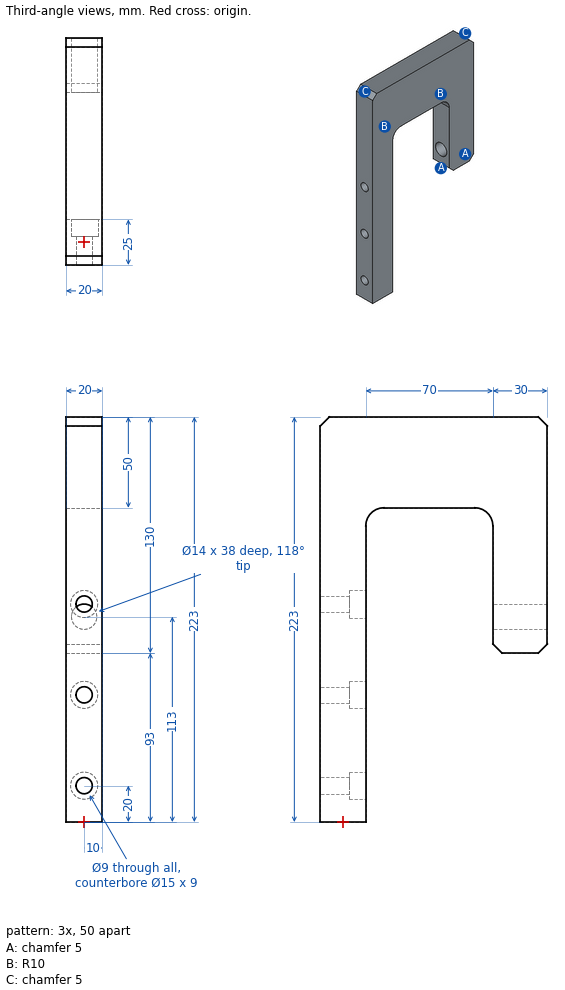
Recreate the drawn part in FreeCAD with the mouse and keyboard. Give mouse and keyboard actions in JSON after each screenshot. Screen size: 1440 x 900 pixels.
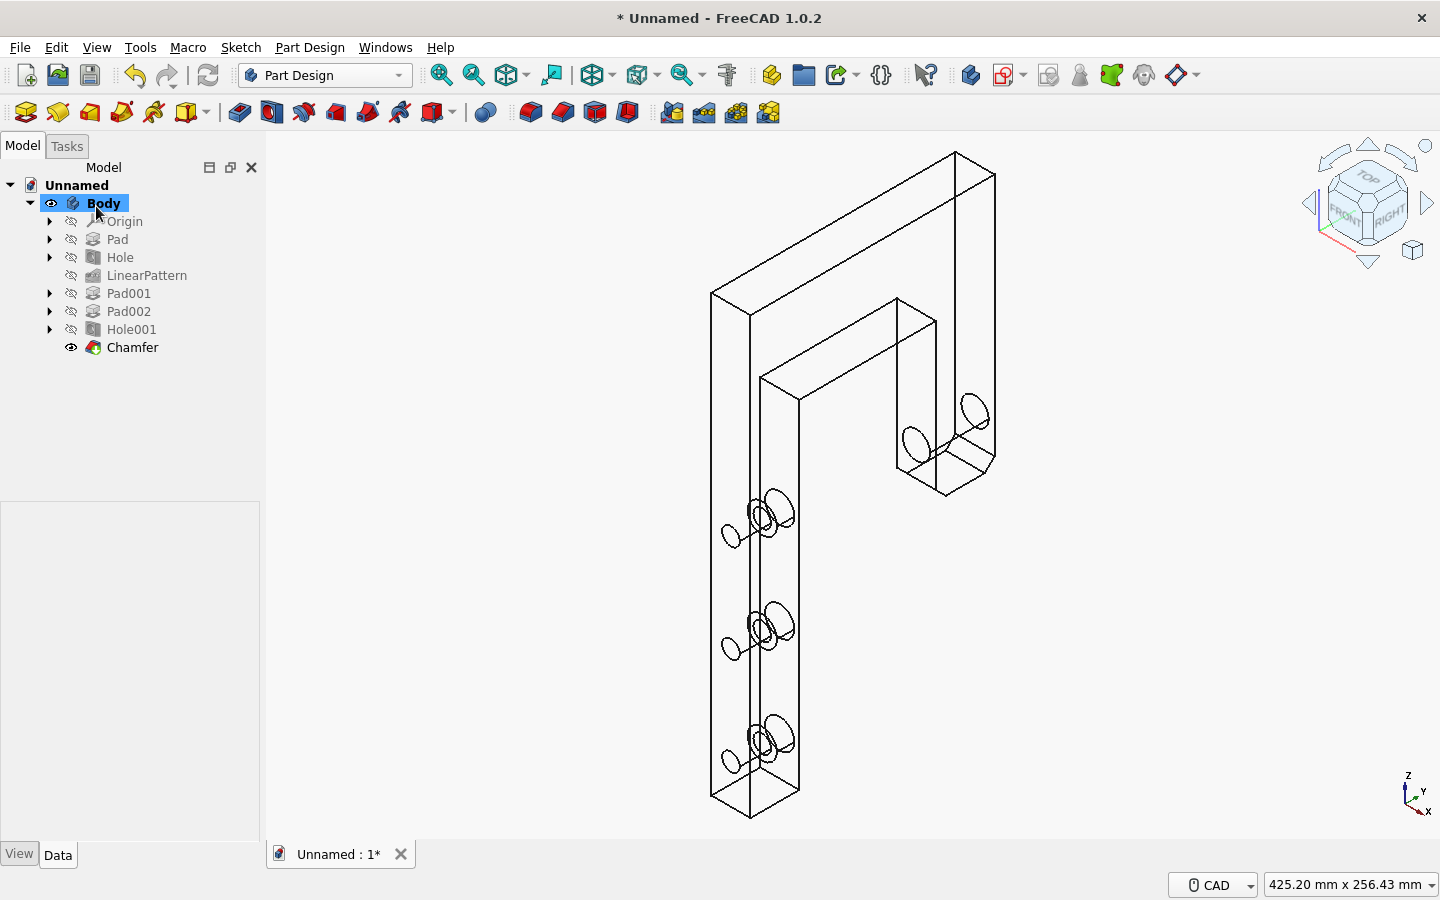
{"action": "left_click", "coordinate": [780, 388]}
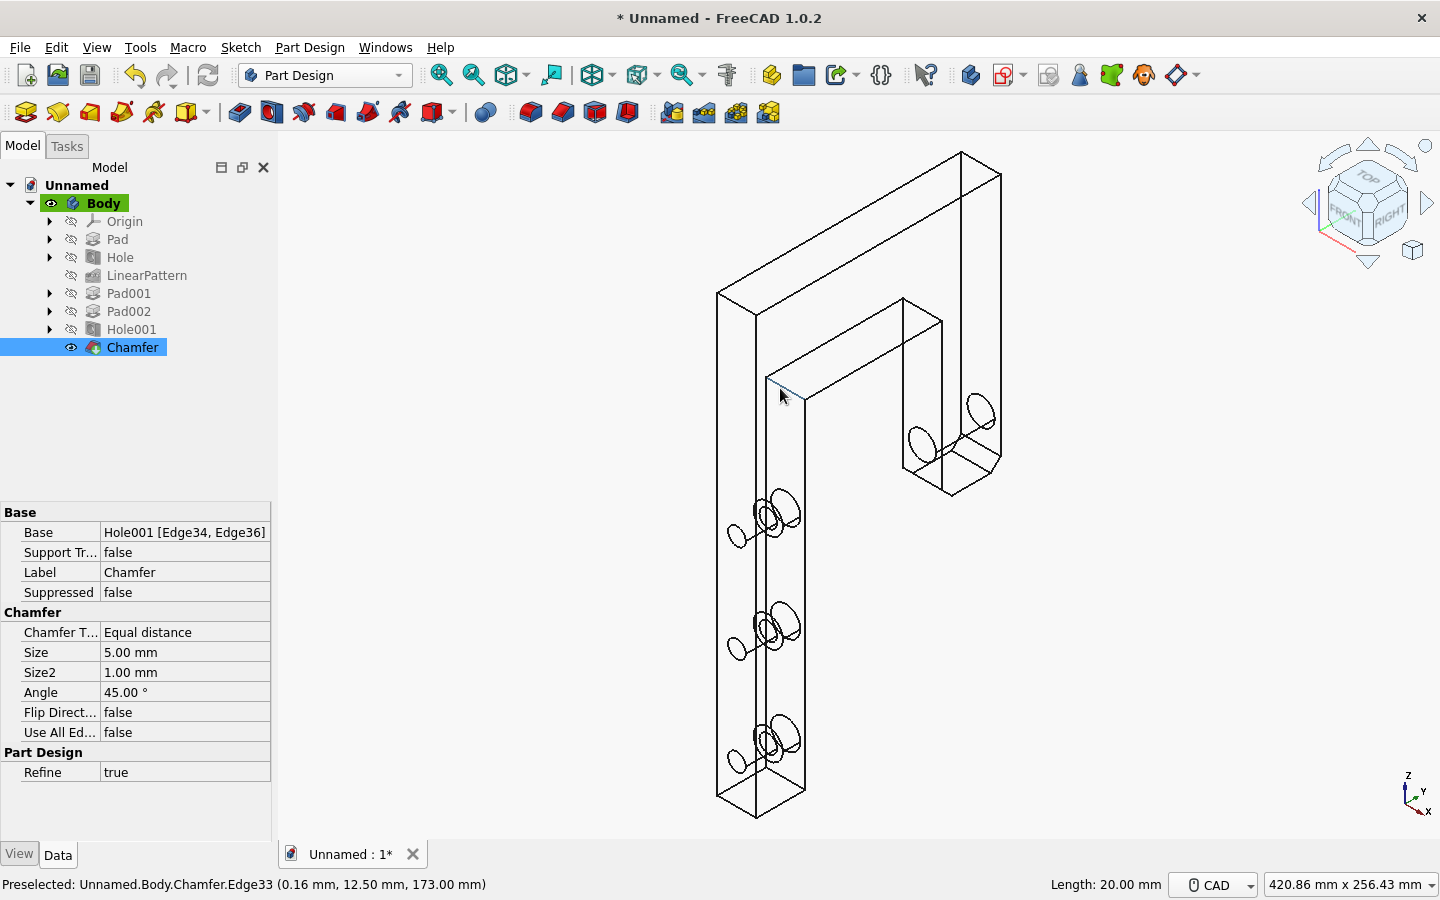
{"action": "left_click", "coordinate": [922, 309], "text": "ctrl"}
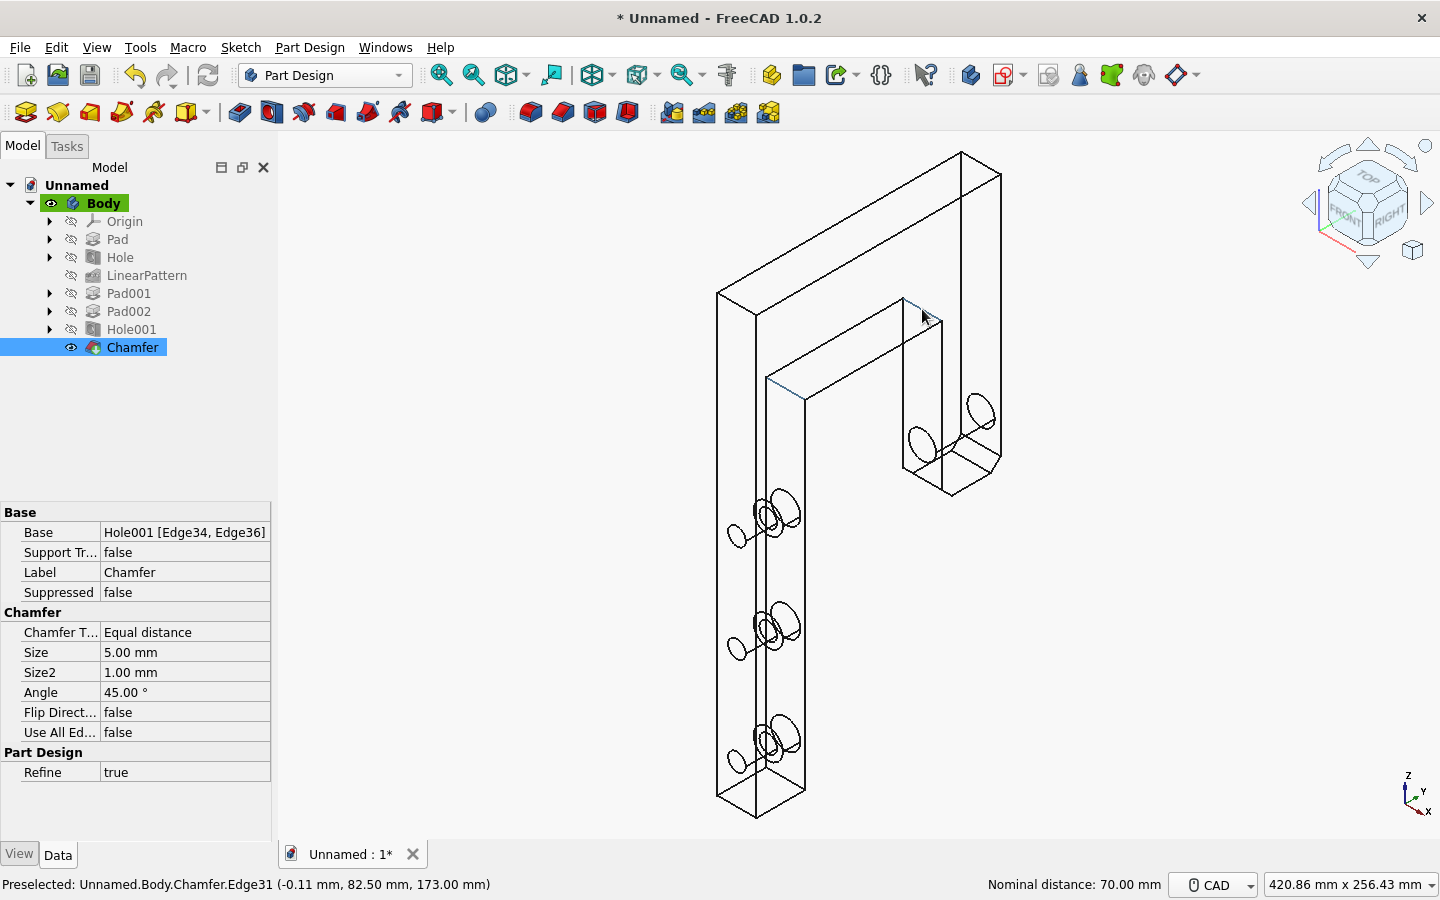
{"action": "key", "text": "v 1"}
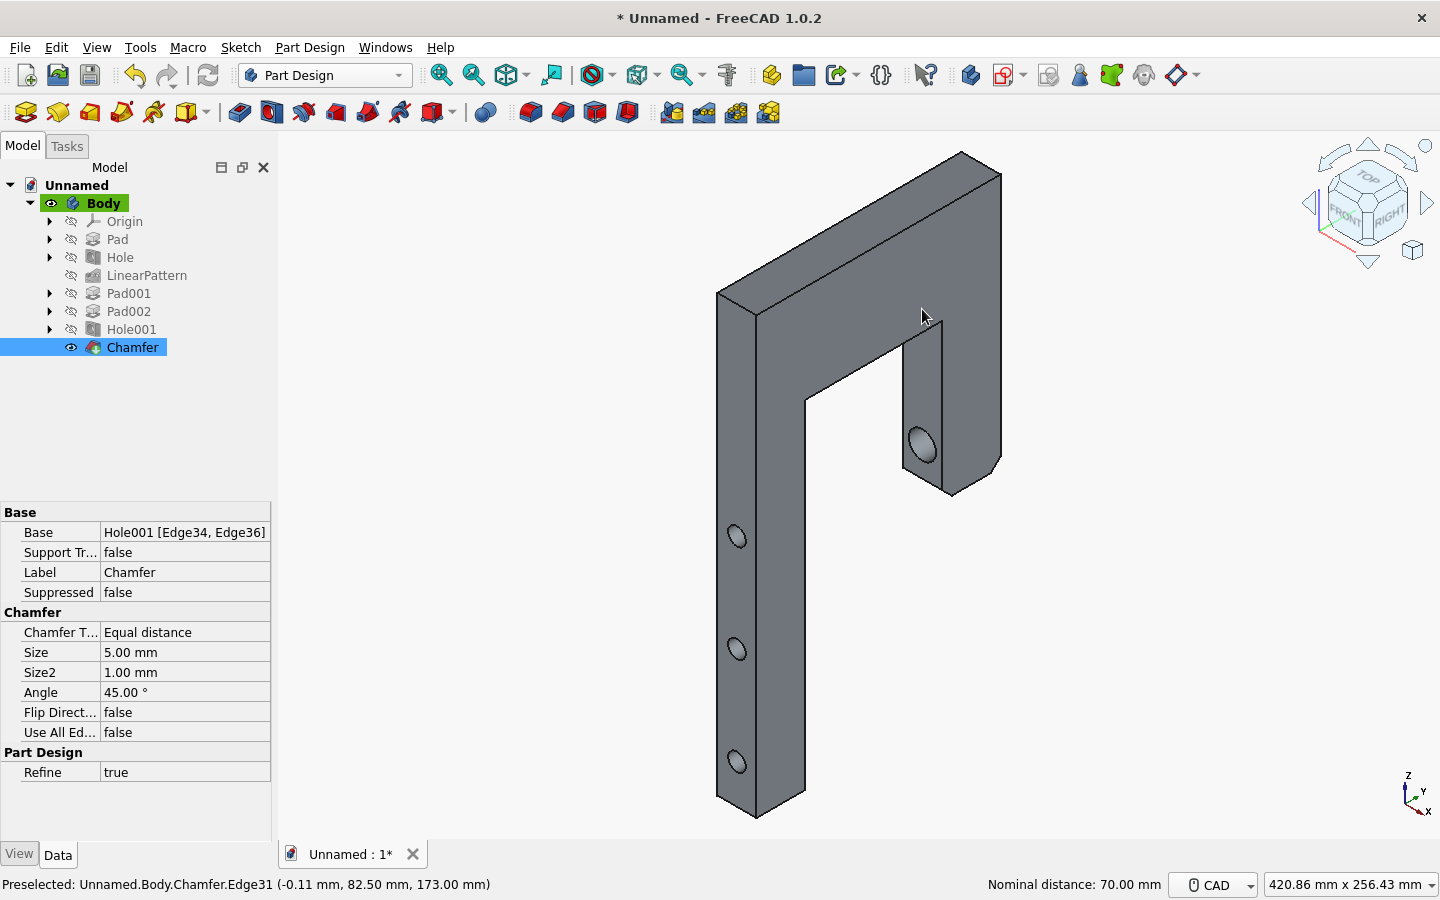
{"action": "left_click", "coordinate": [532, 112]}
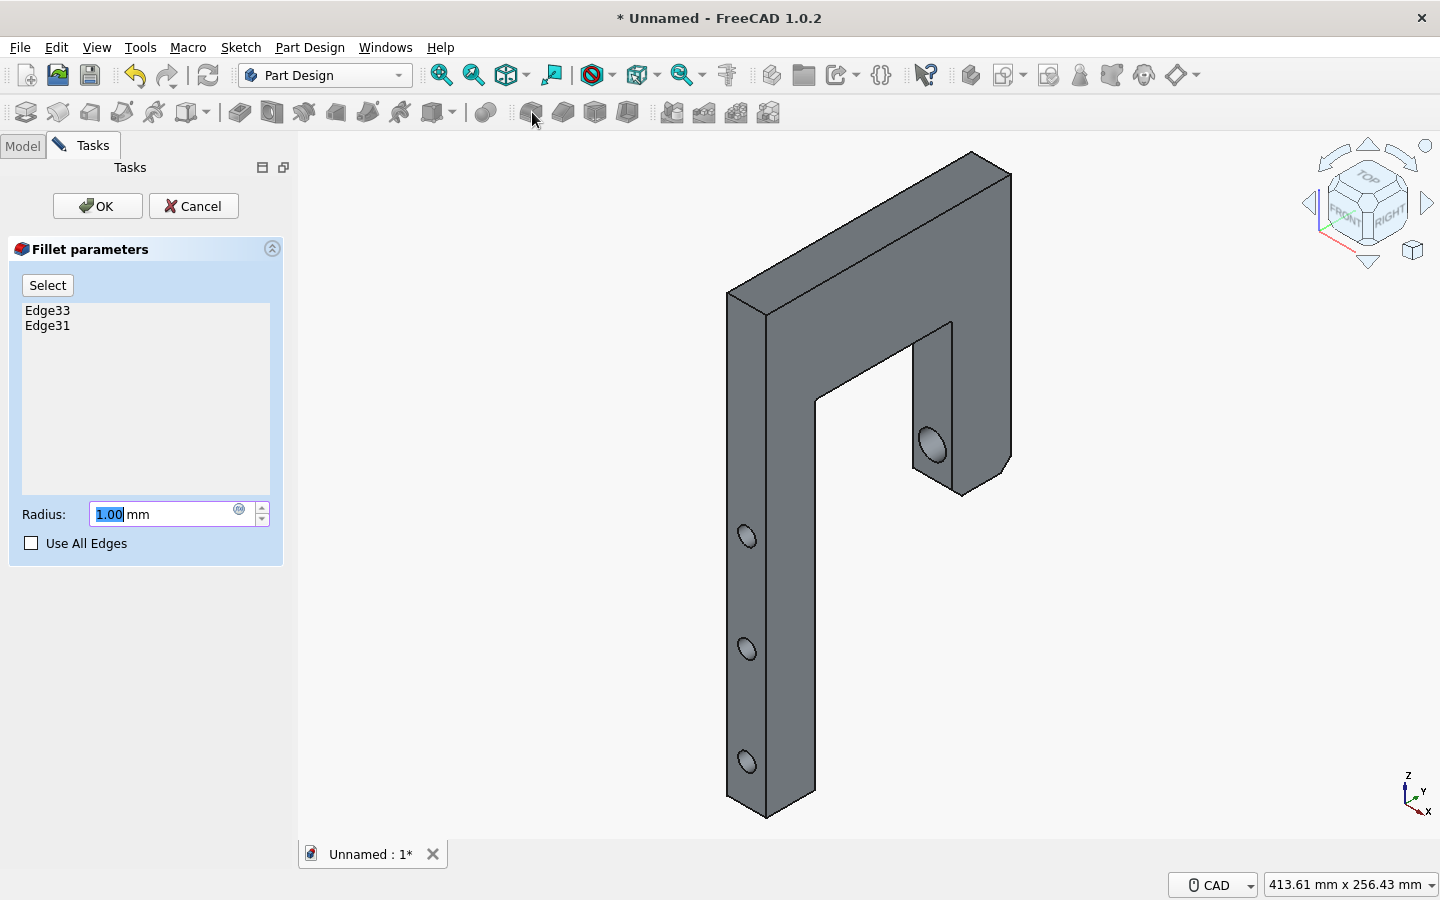
{"action": "type", "text": "10"}
{"action": "key", "text": "Tab"}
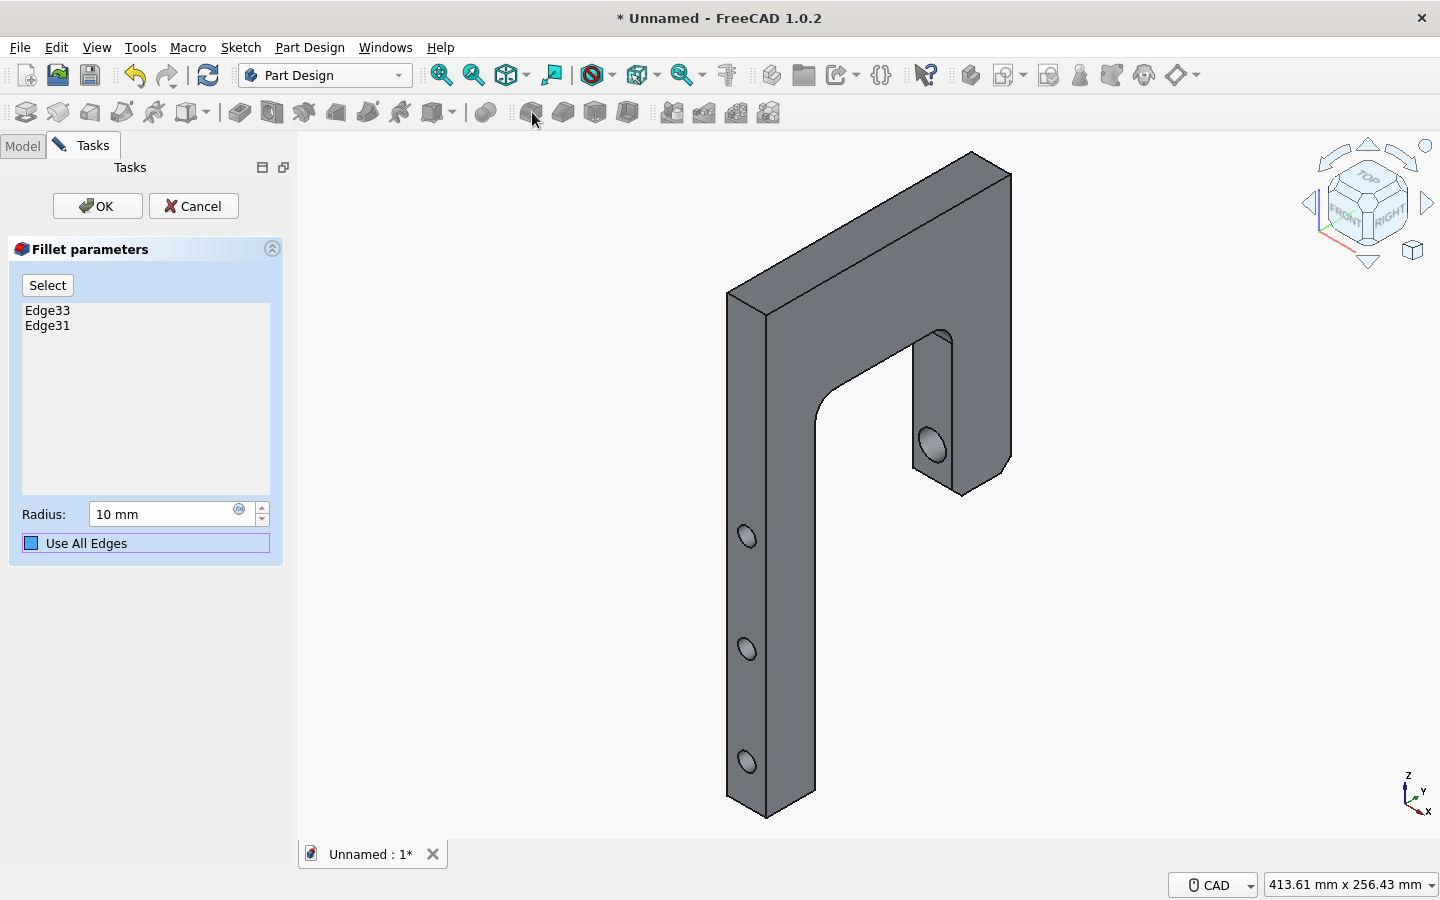
{"action": "left_click", "coordinate": [98, 206]}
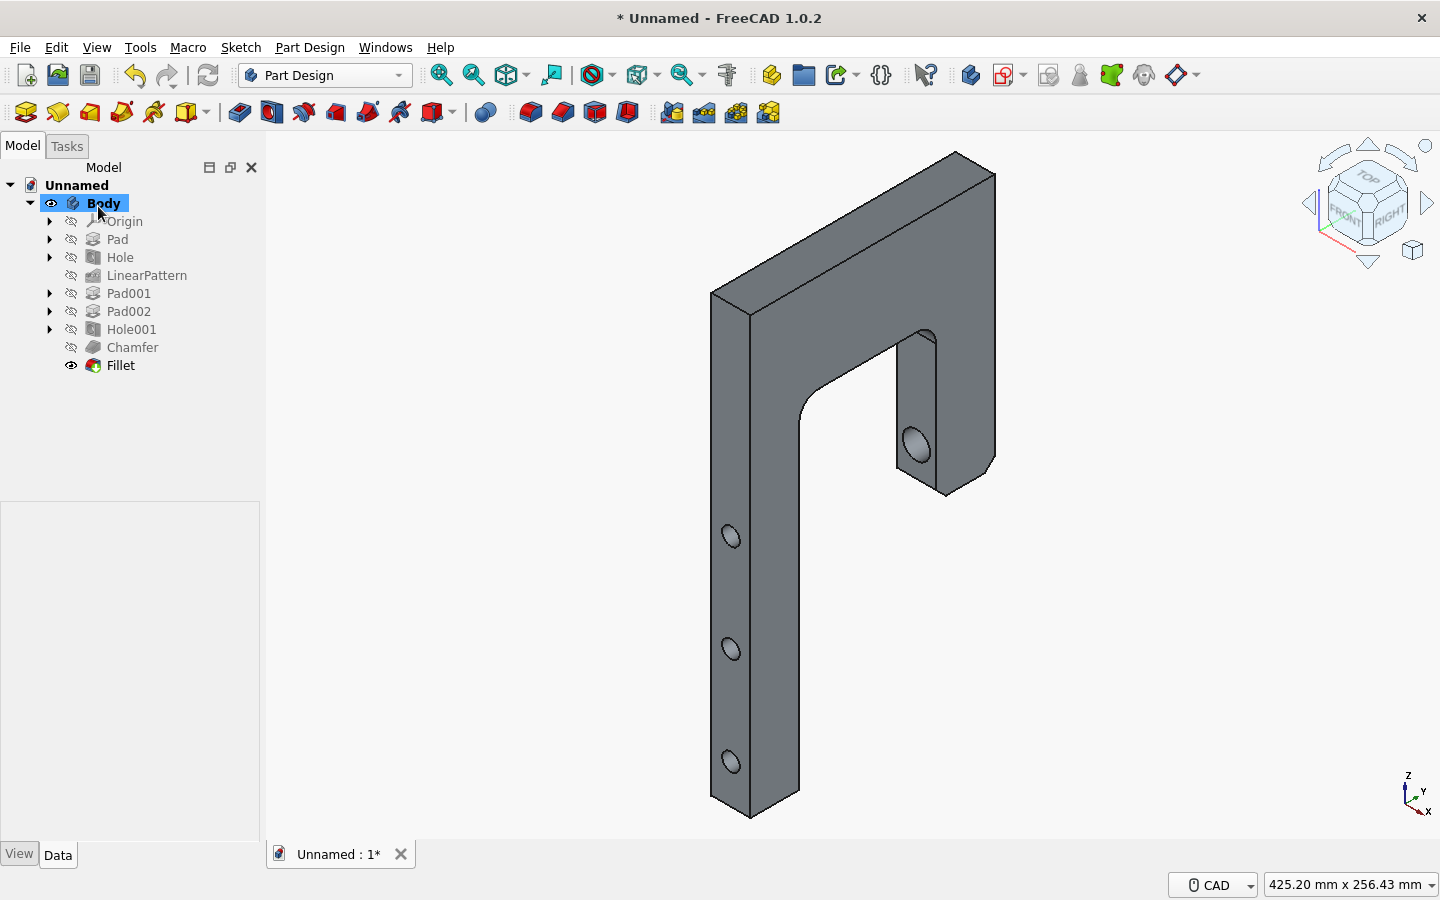
{"action": "left_click", "coordinate": [731, 303]}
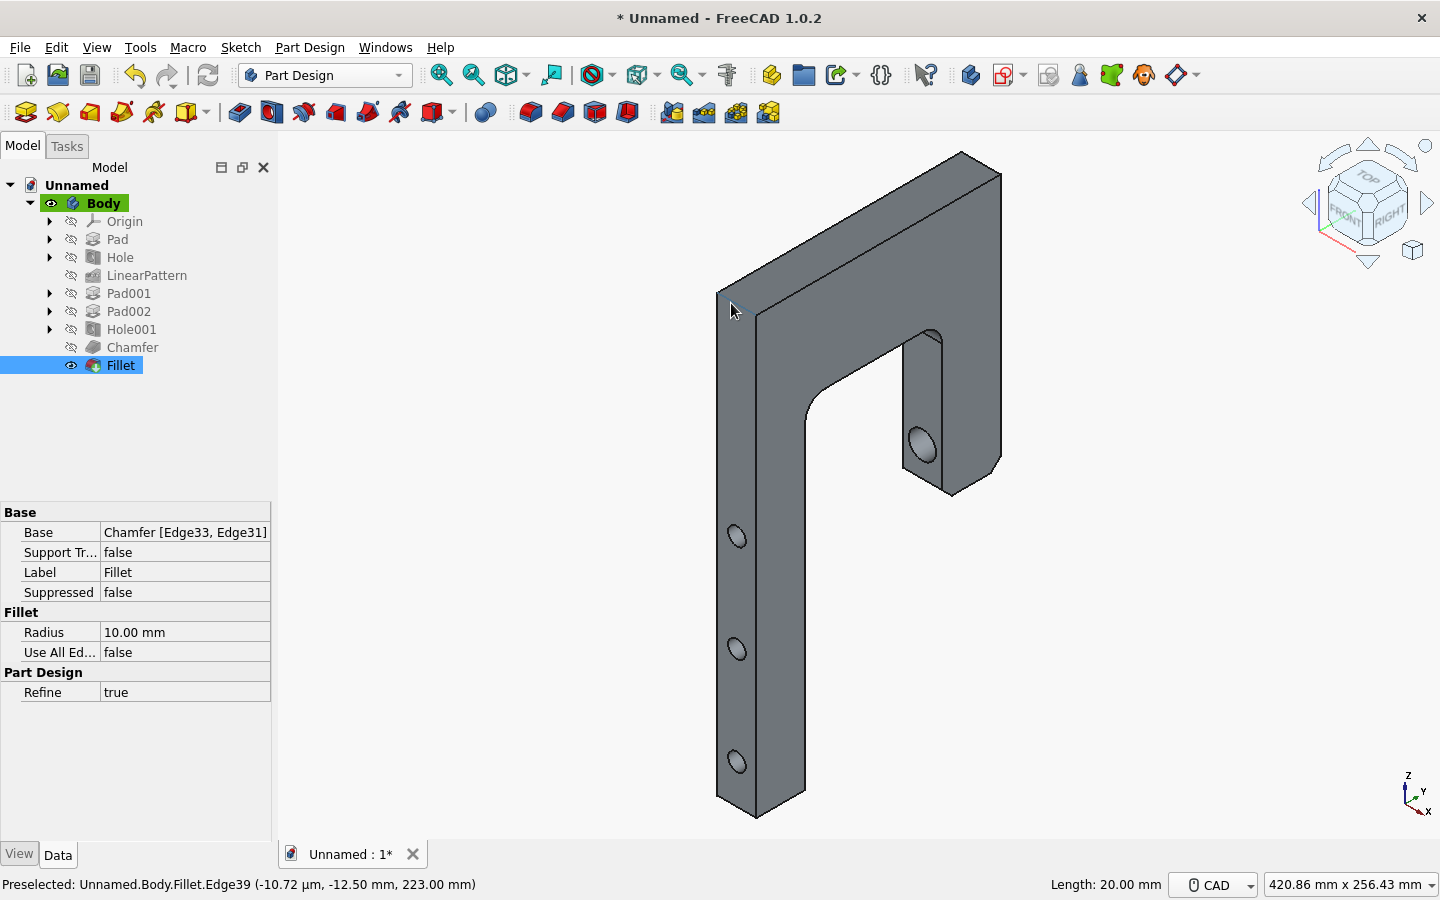
{"action": "key", "text": "2"}